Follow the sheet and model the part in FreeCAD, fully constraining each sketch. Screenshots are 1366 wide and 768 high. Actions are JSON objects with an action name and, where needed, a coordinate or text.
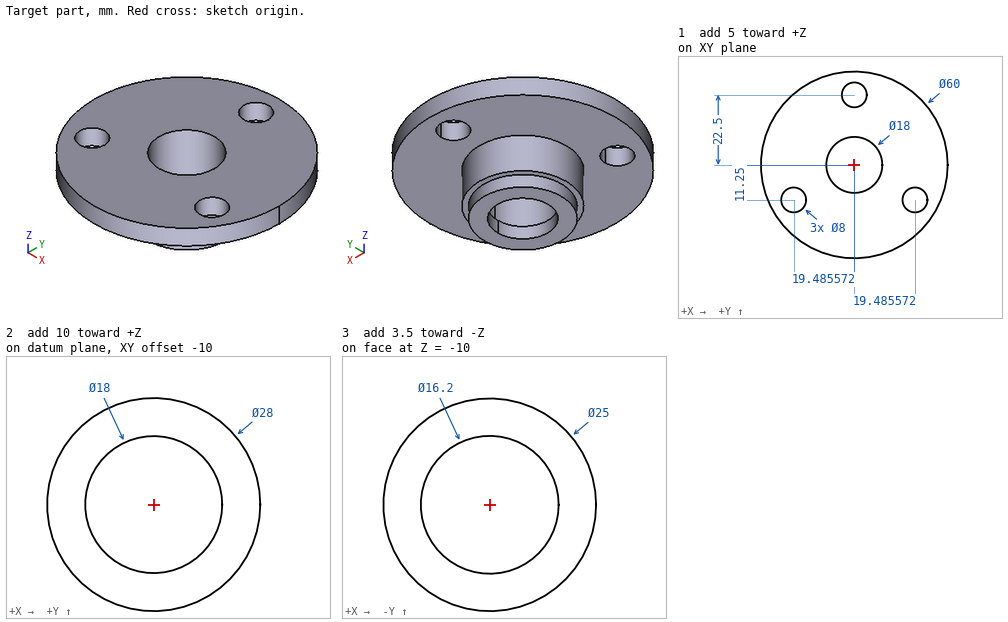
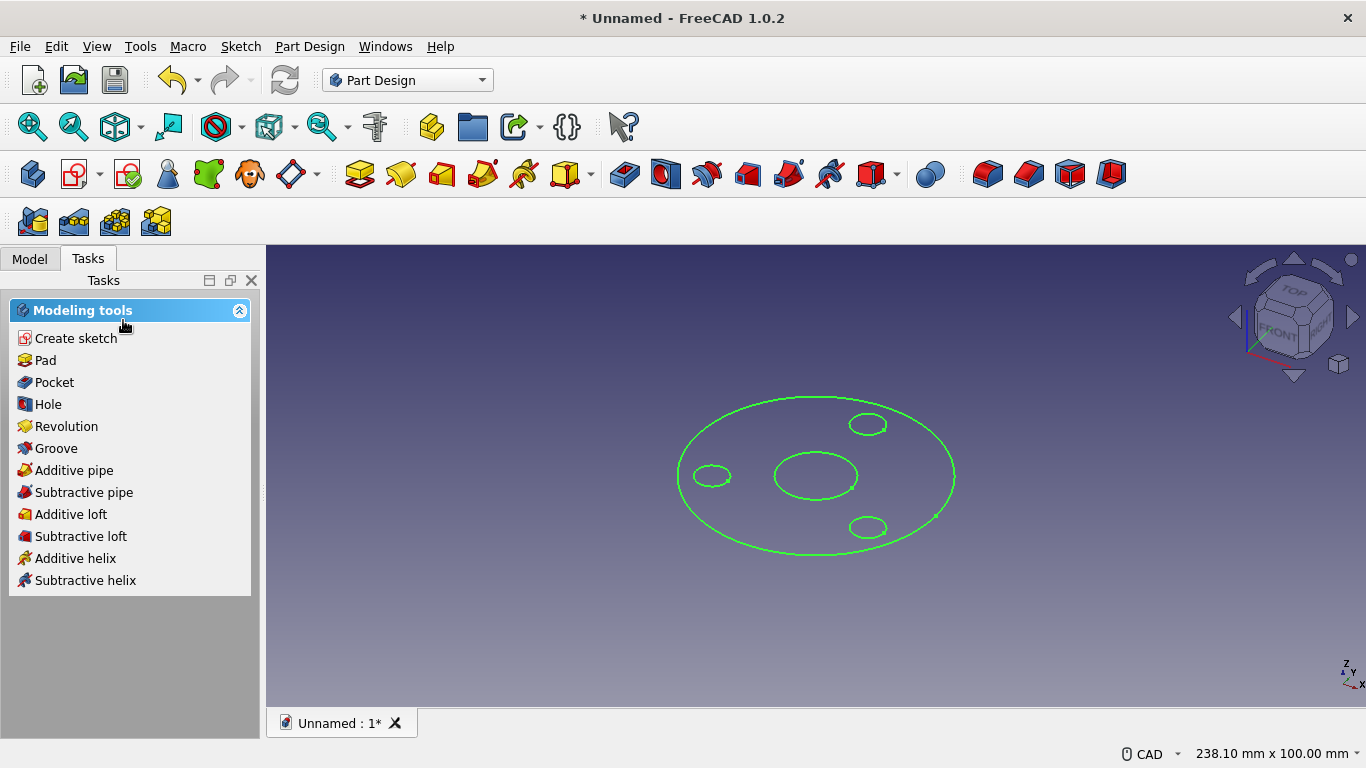
{"action": "left_click", "coordinate": [360, 174]}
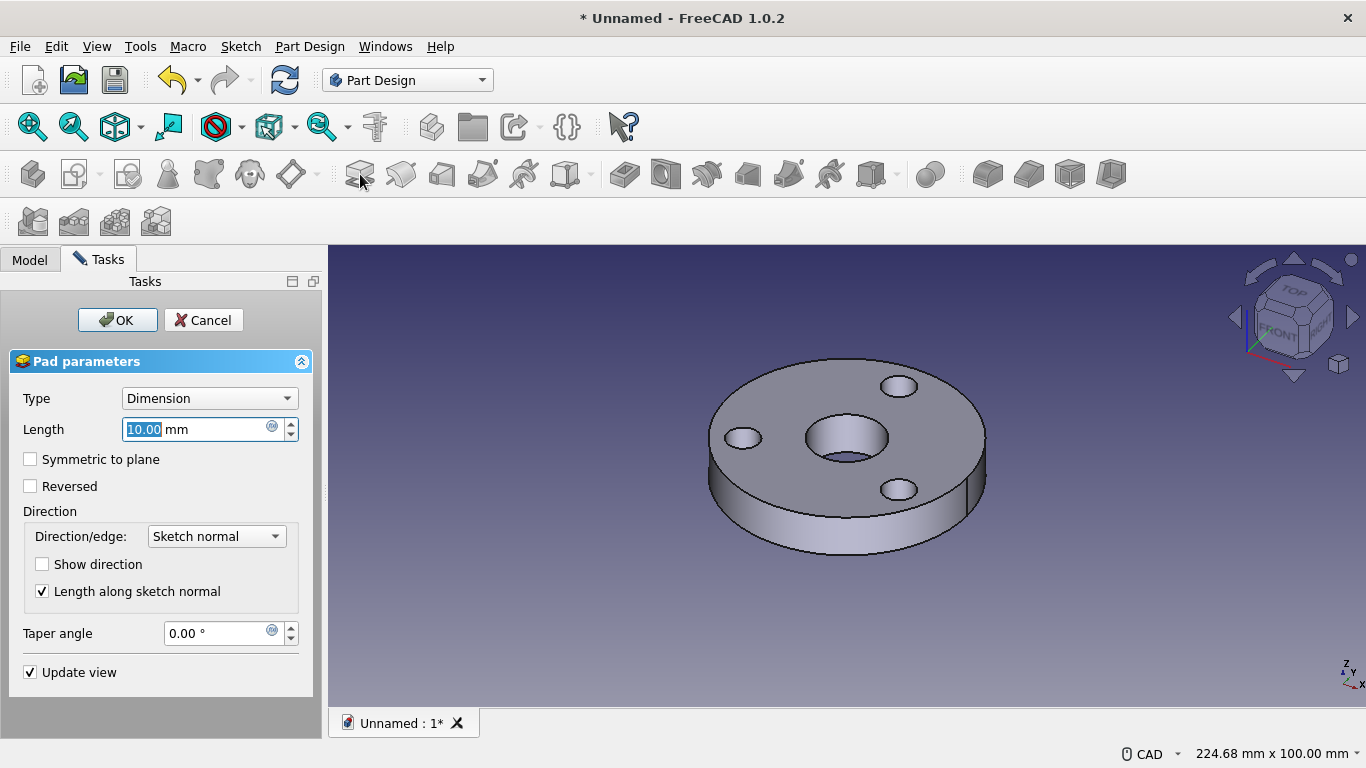
{"action": "type", "text": "5"}
{"action": "key", "text": "Tab"}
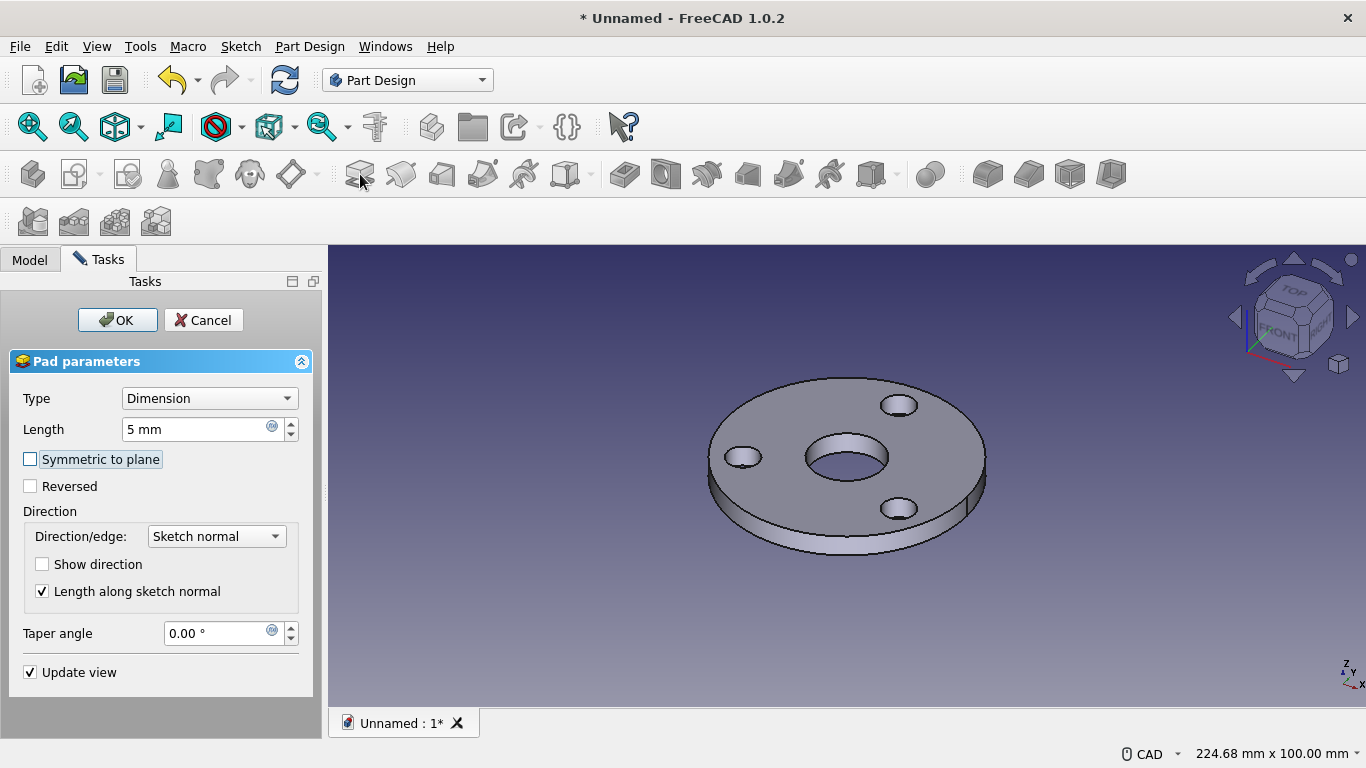
{"action": "left_click", "coordinate": [118, 320]}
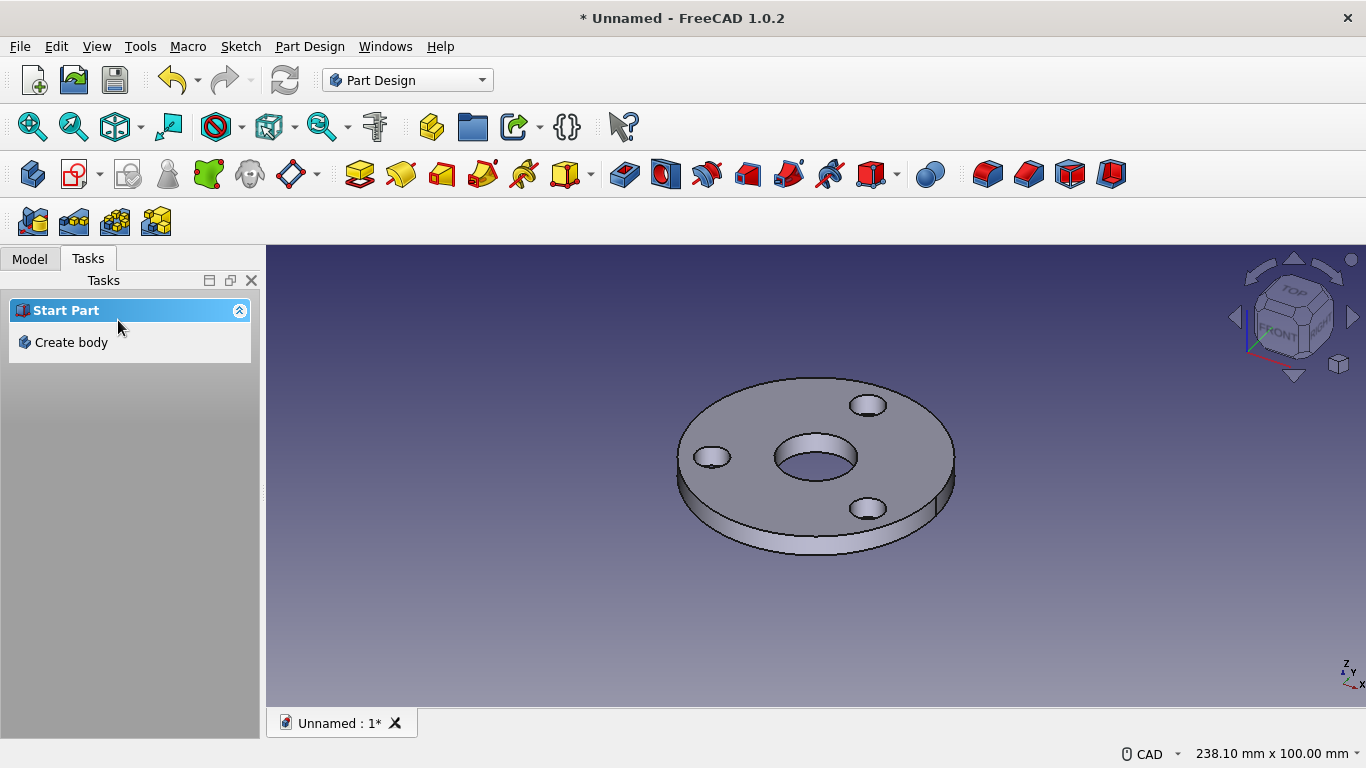
{"action": "left_click", "coordinate": [30, 258]}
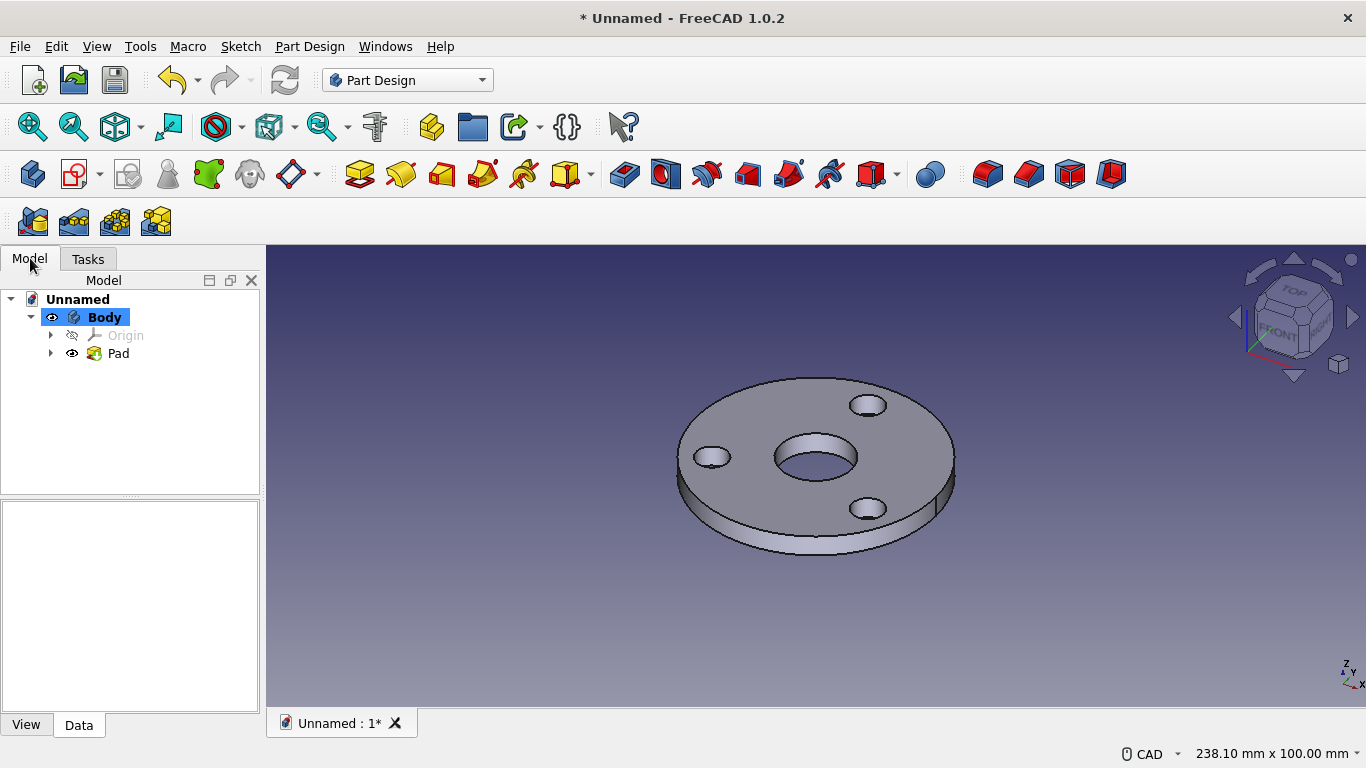
{"action": "left_click", "coordinate": [51, 335]}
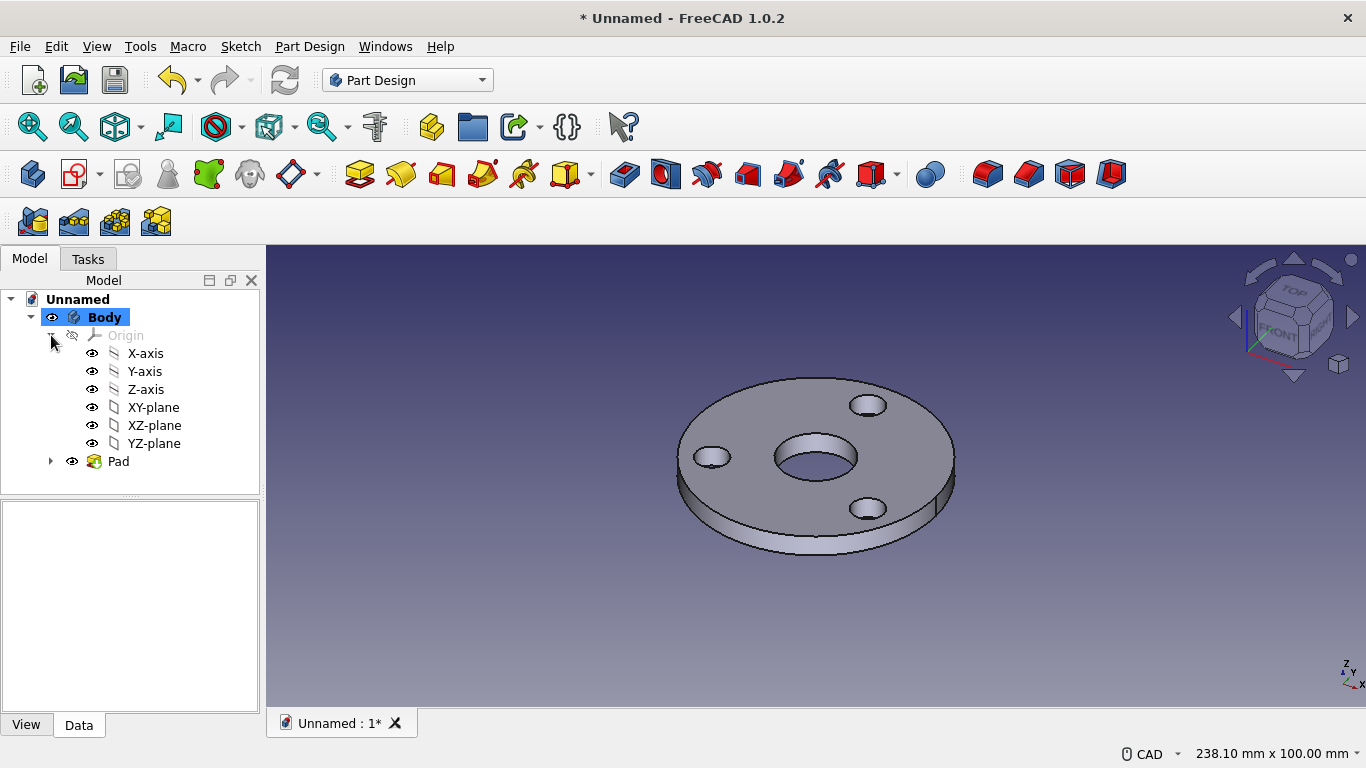
{"action": "left_click", "coordinate": [137, 407]}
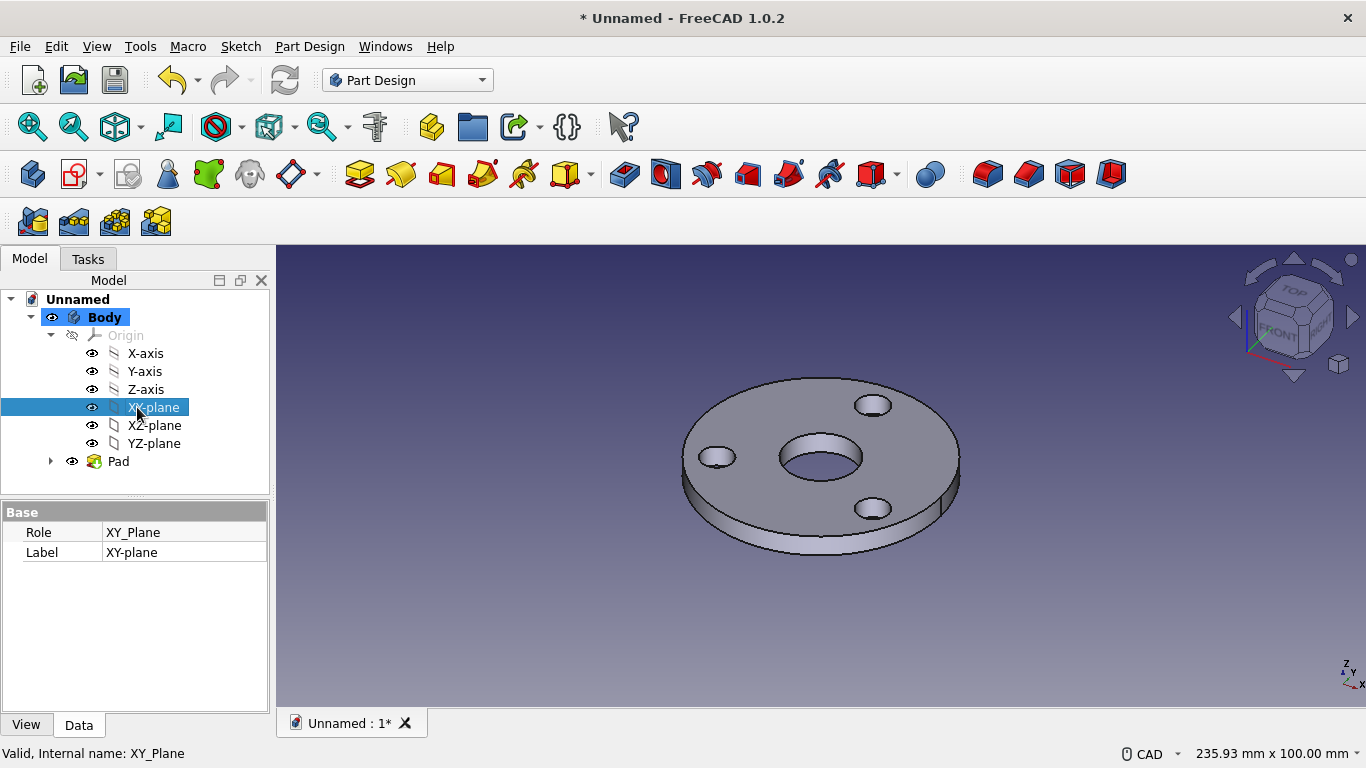
{"action": "left_click", "coordinate": [290, 174]}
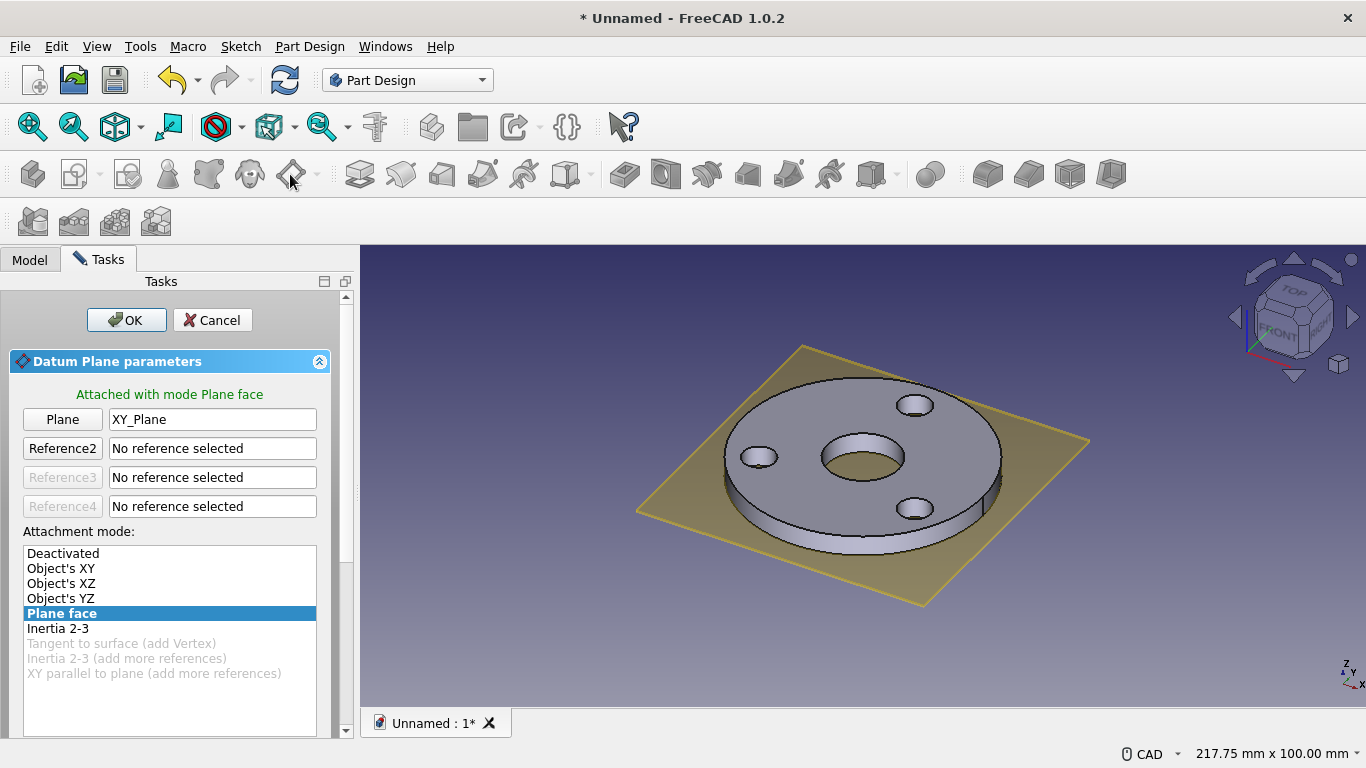
{"action": "scroll", "coordinate": [346, 514], "scroll_direction": "down", "scroll_amount": 4}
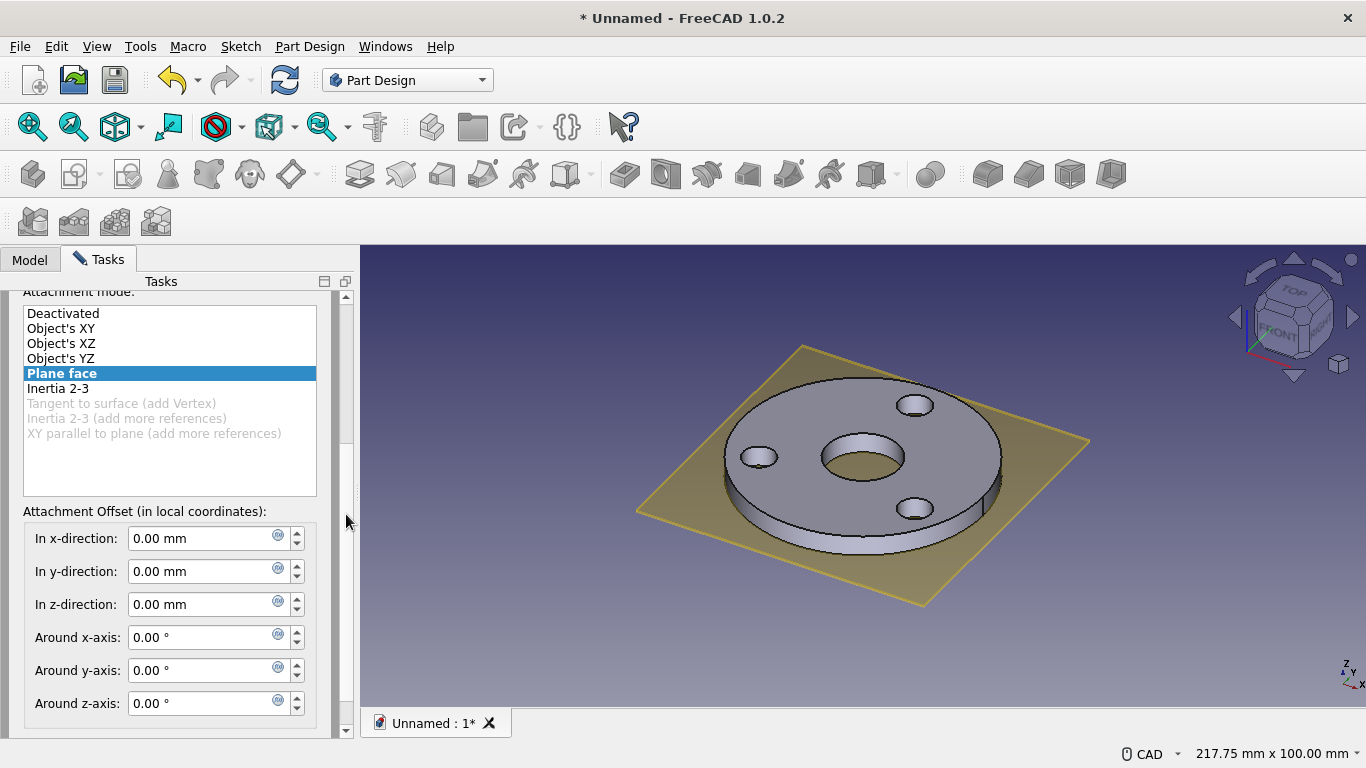
{"action": "triple_click", "coordinate": [210, 604]}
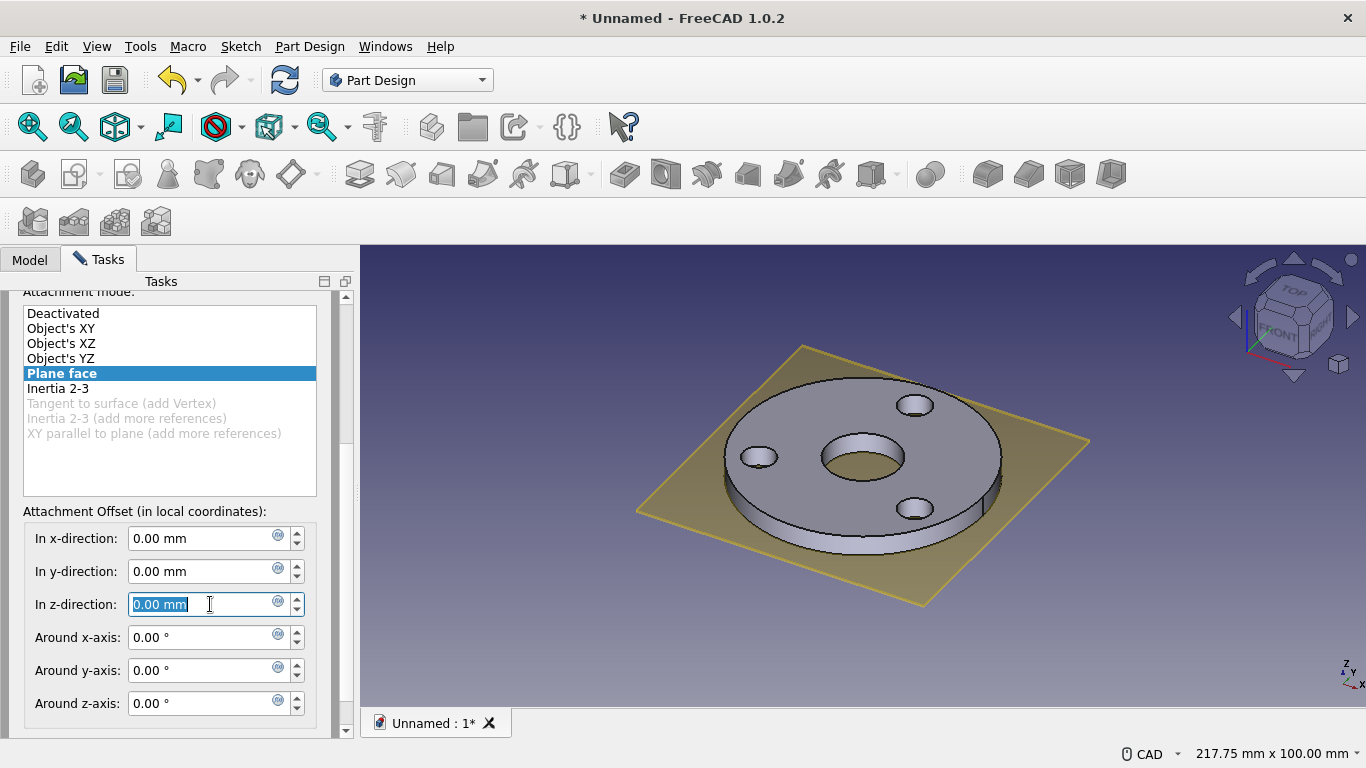
{"action": "type", "text": "-10"}
{"action": "key", "text": "Tab"}